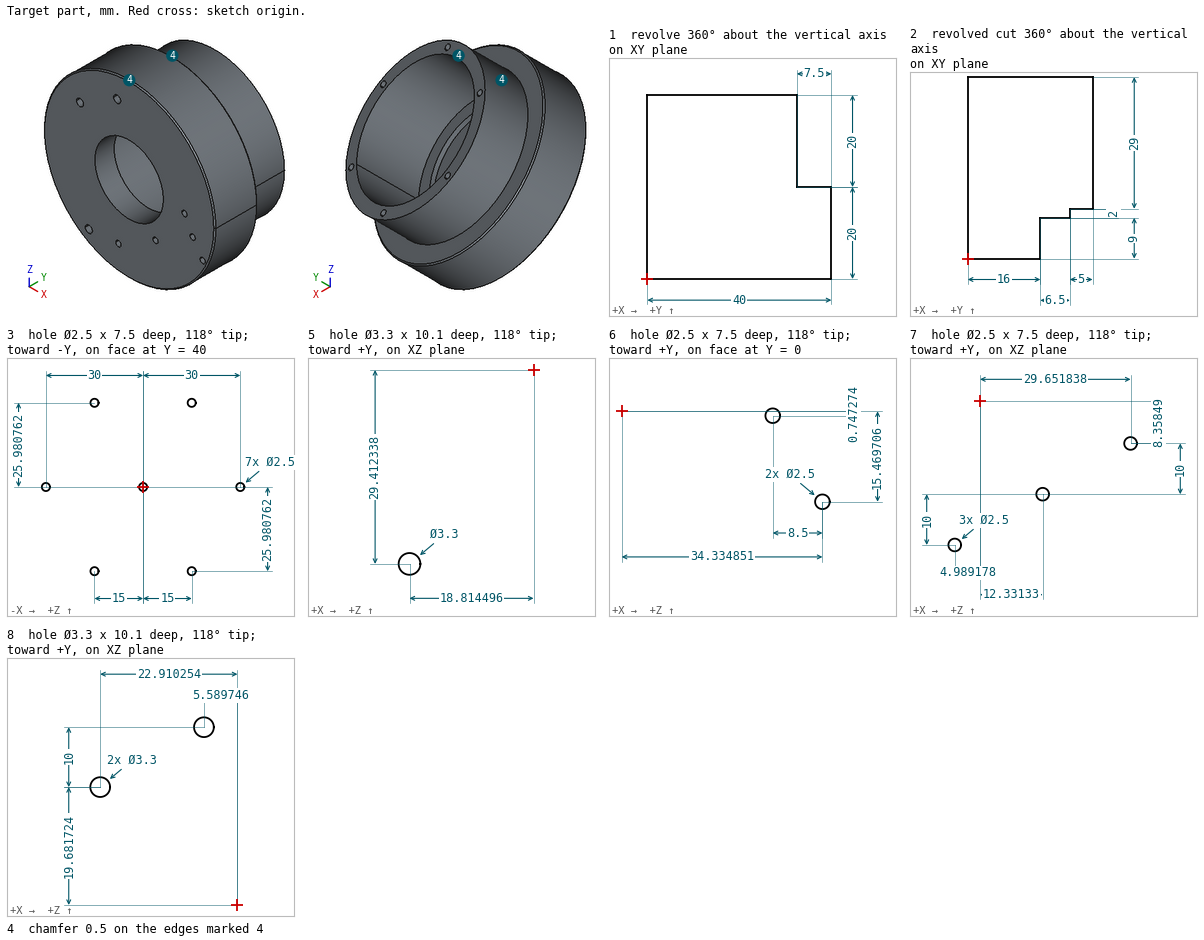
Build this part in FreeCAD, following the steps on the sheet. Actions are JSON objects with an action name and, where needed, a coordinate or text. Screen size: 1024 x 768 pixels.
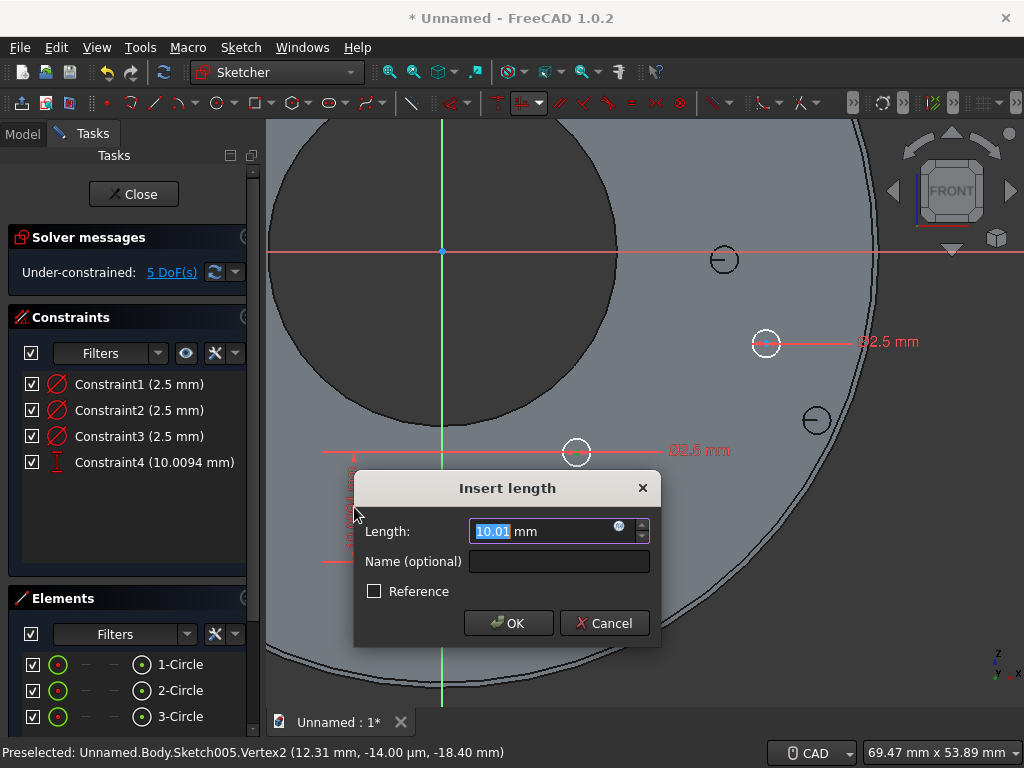
{"action": "type", "text": "10"}
{"action": "key", "text": "Return"}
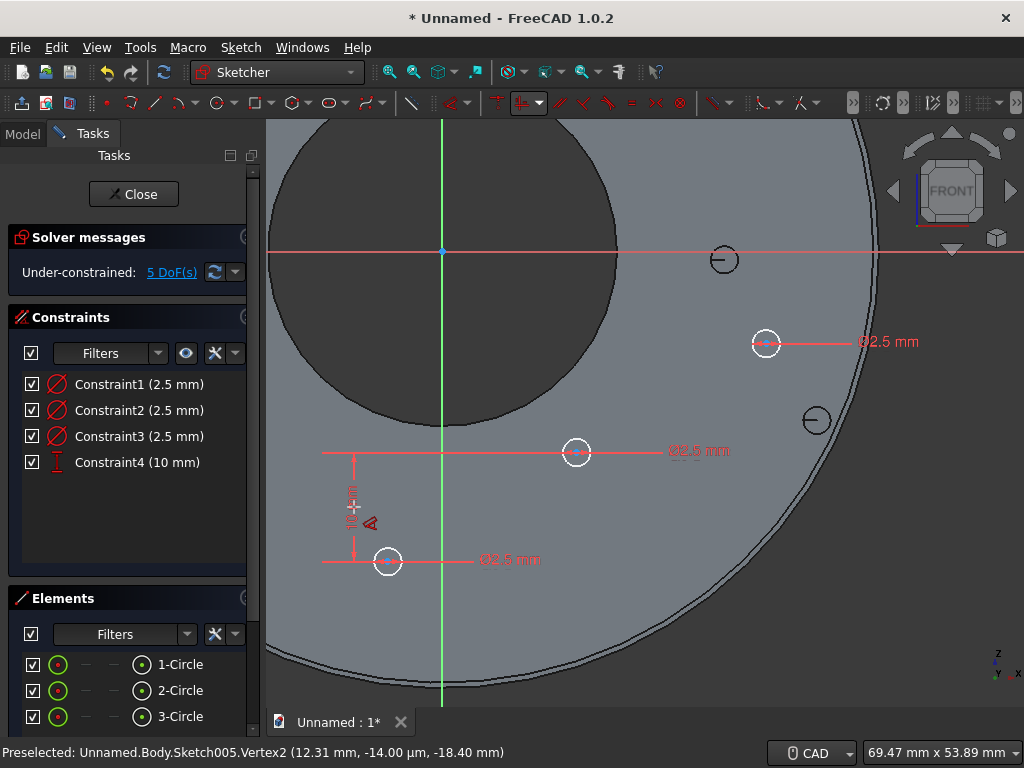
{"action": "left_click", "coordinate": [577, 453]}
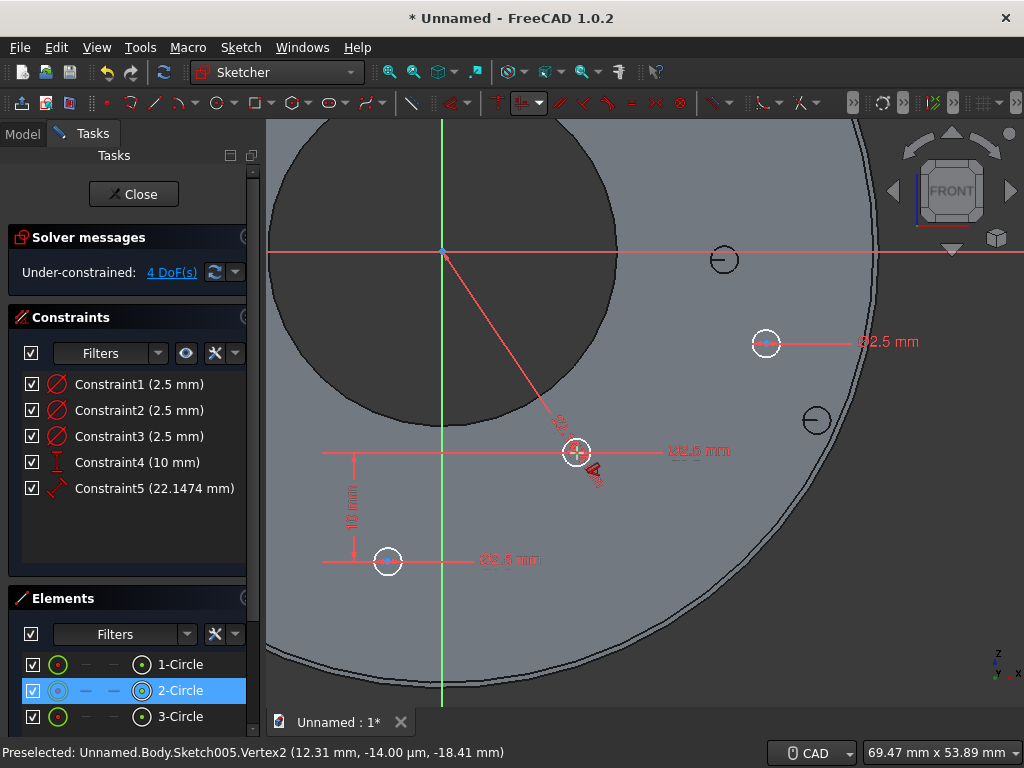
{"action": "left_click", "coordinate": [766, 344]}
{"action": "left_click", "coordinate": [800, 398]}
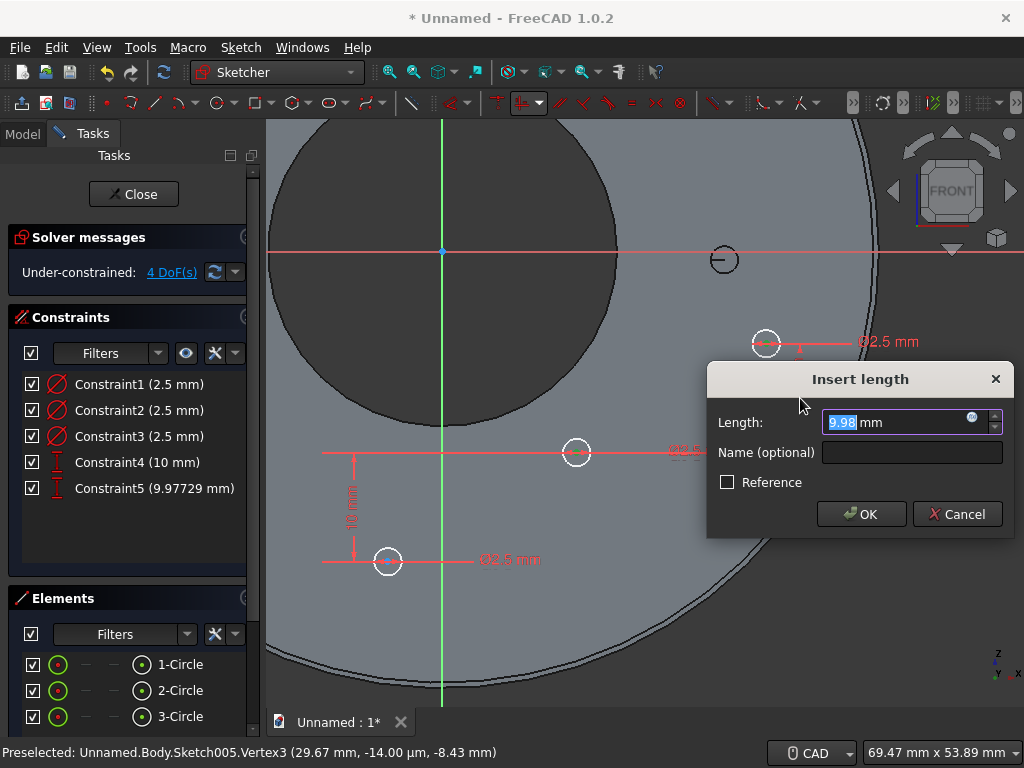
{"action": "type", "text": "10"}
{"action": "key", "text": "Return"}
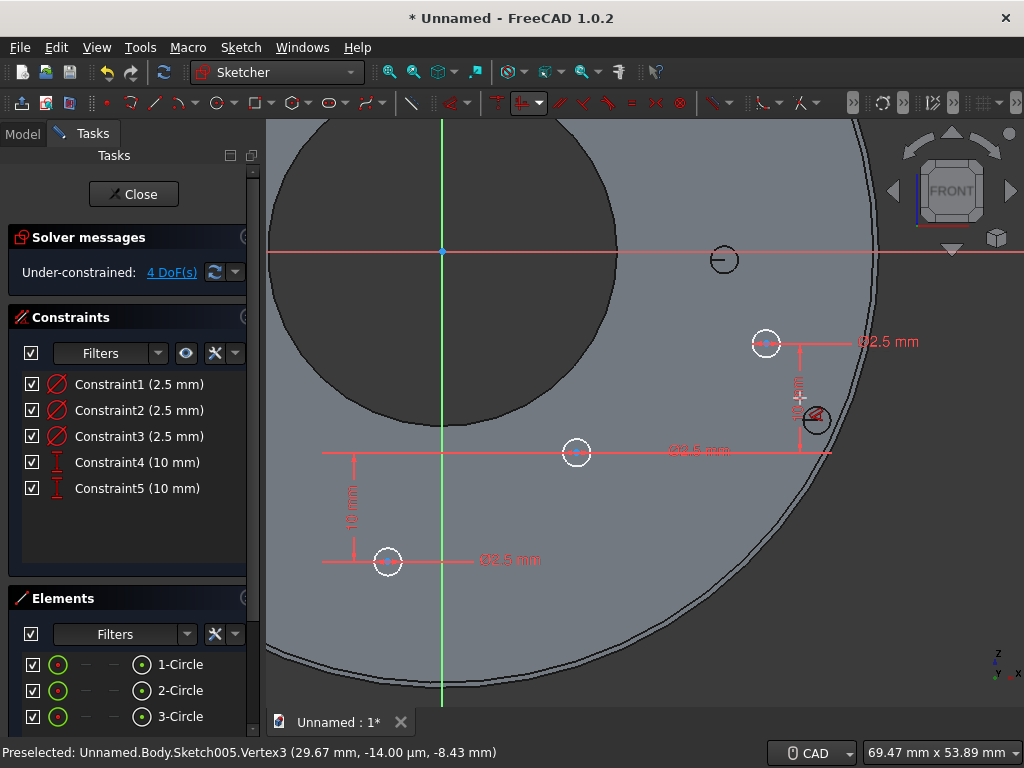
{"action": "left_click", "coordinate": [766, 344]}
{"action": "left_click", "coordinate": [800, 298]}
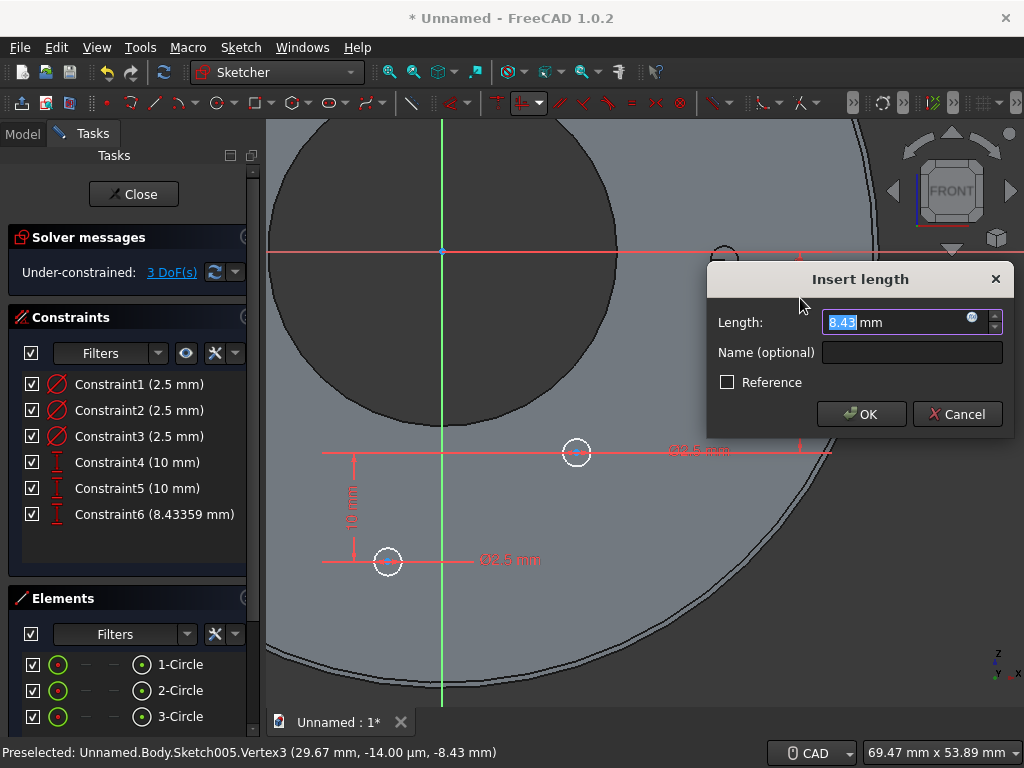
{"action": "type", "text": "8.35849"}
{"action": "key", "text": "Return"}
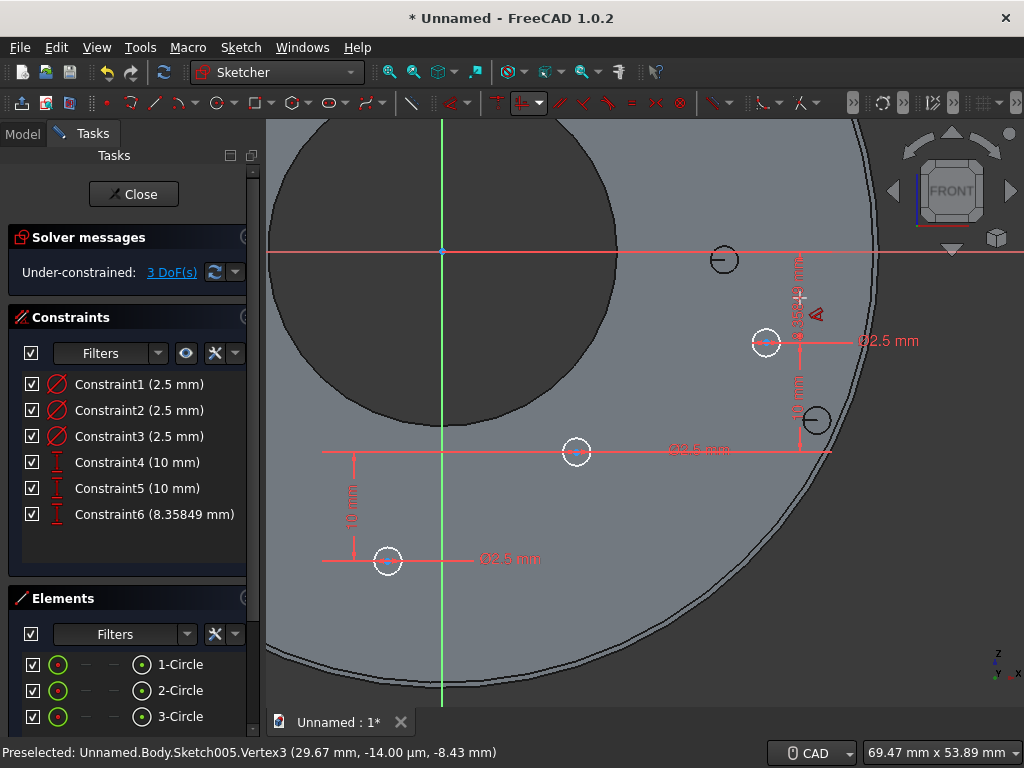
{"action": "left_click", "coordinate": [388, 561]}
{"action": "left_click", "coordinate": [415, 218]}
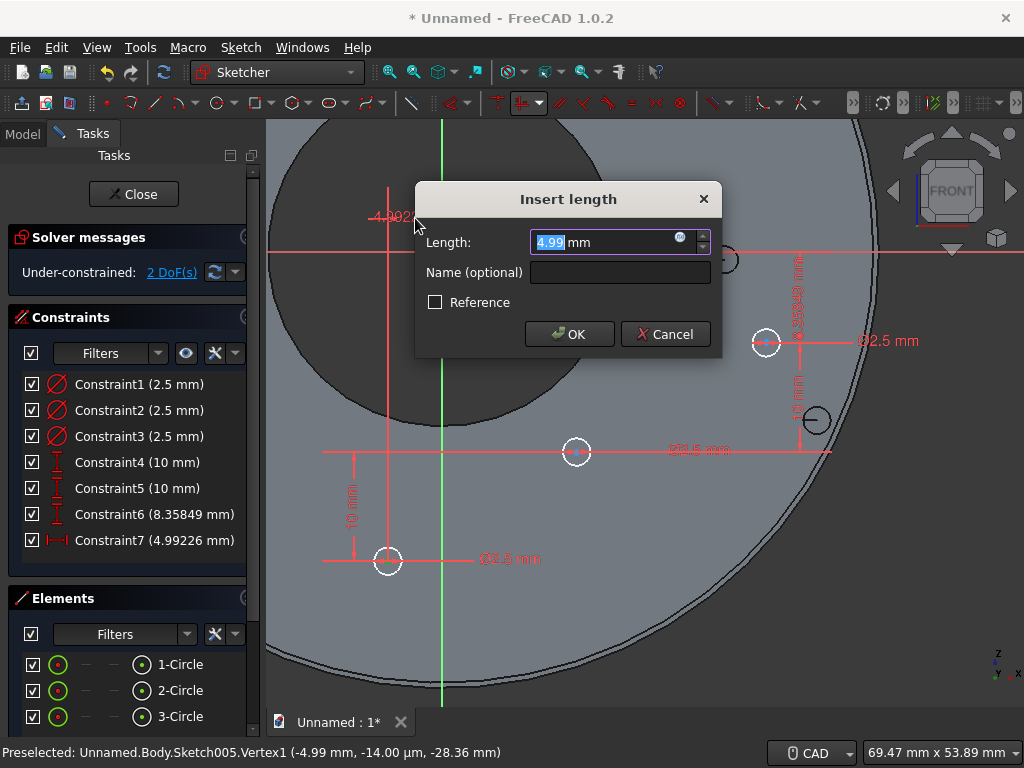
{"action": "type", "text": "4.989178"}
{"action": "key", "text": "Return"}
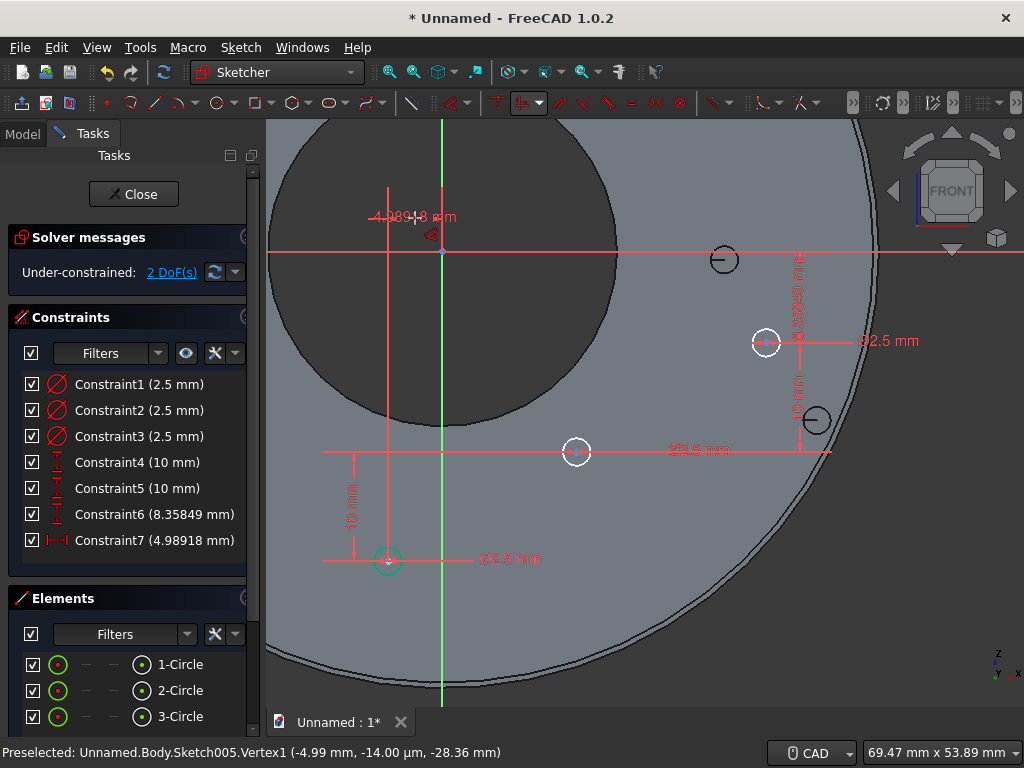
{"action": "left_click", "coordinate": [577, 452]}
{"action": "left_click", "coordinate": [510, 218]}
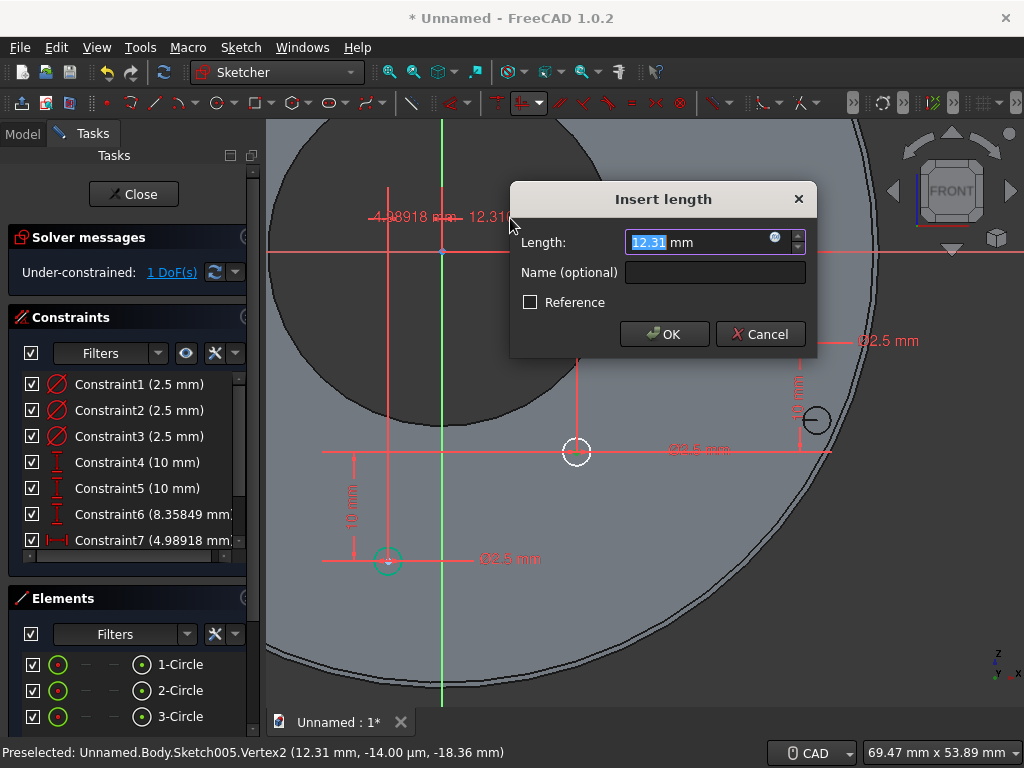
{"action": "type", "text": "12.33133"}
{"action": "key", "text": "Return"}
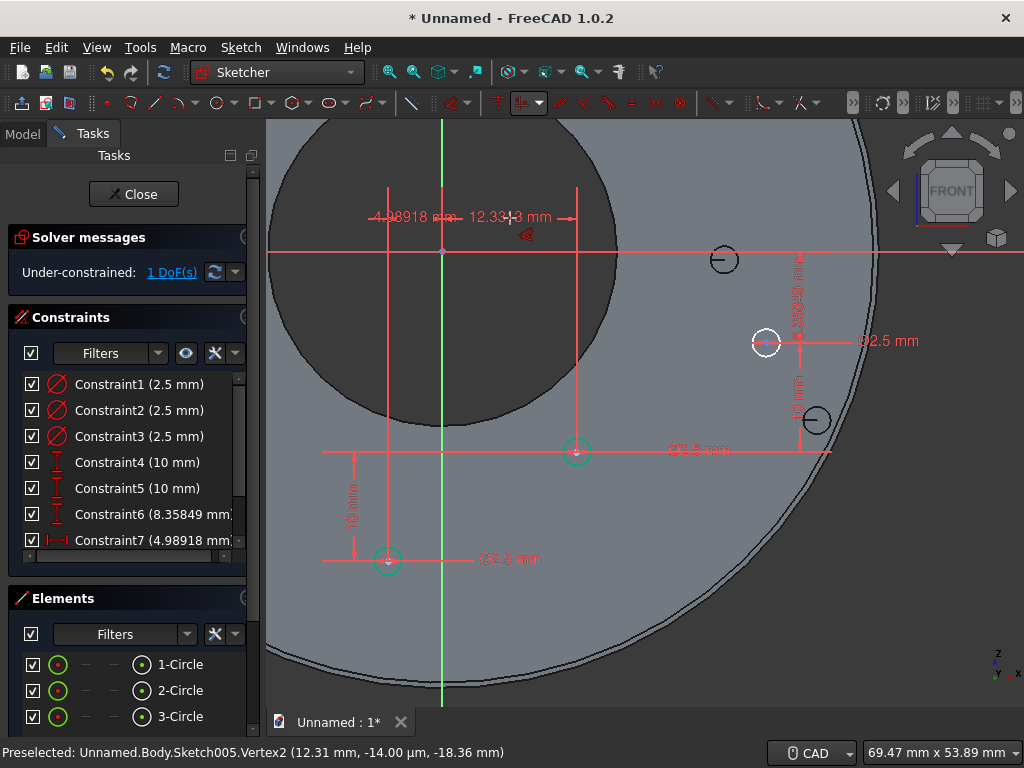
{"action": "left_click", "coordinate": [766, 343]}
{"action": "left_click", "coordinate": [604, 218]}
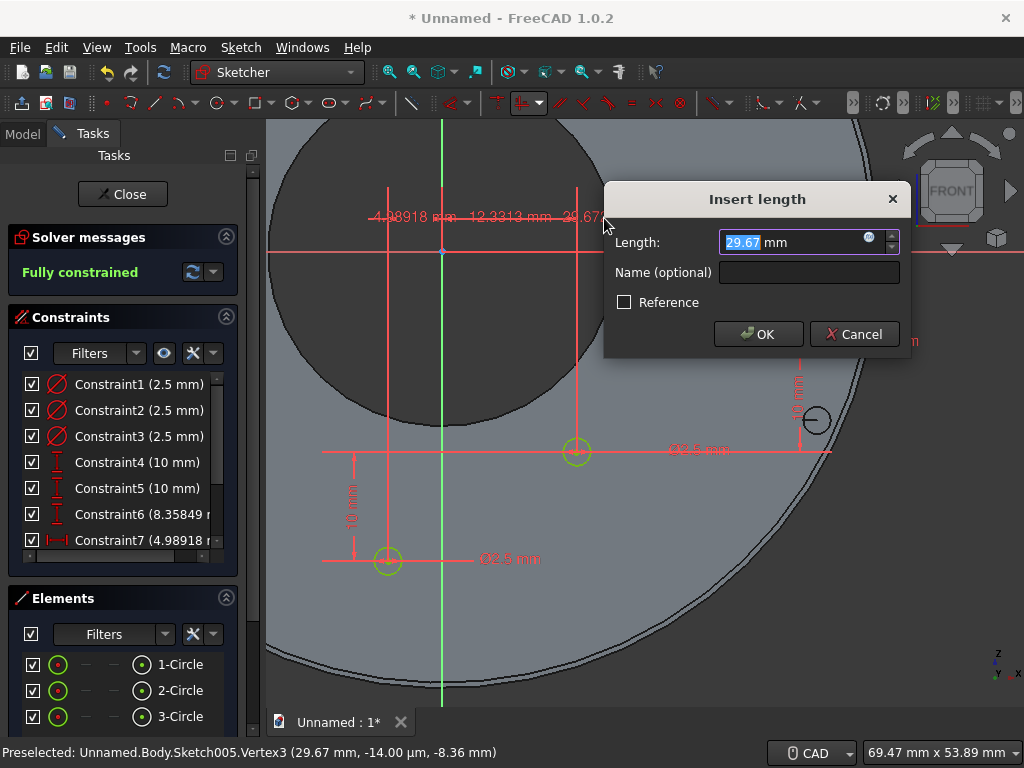
{"action": "type", "text": "29.651838"}
{"action": "key", "text": "Return"}
{"action": "key", "text": "Escape"}